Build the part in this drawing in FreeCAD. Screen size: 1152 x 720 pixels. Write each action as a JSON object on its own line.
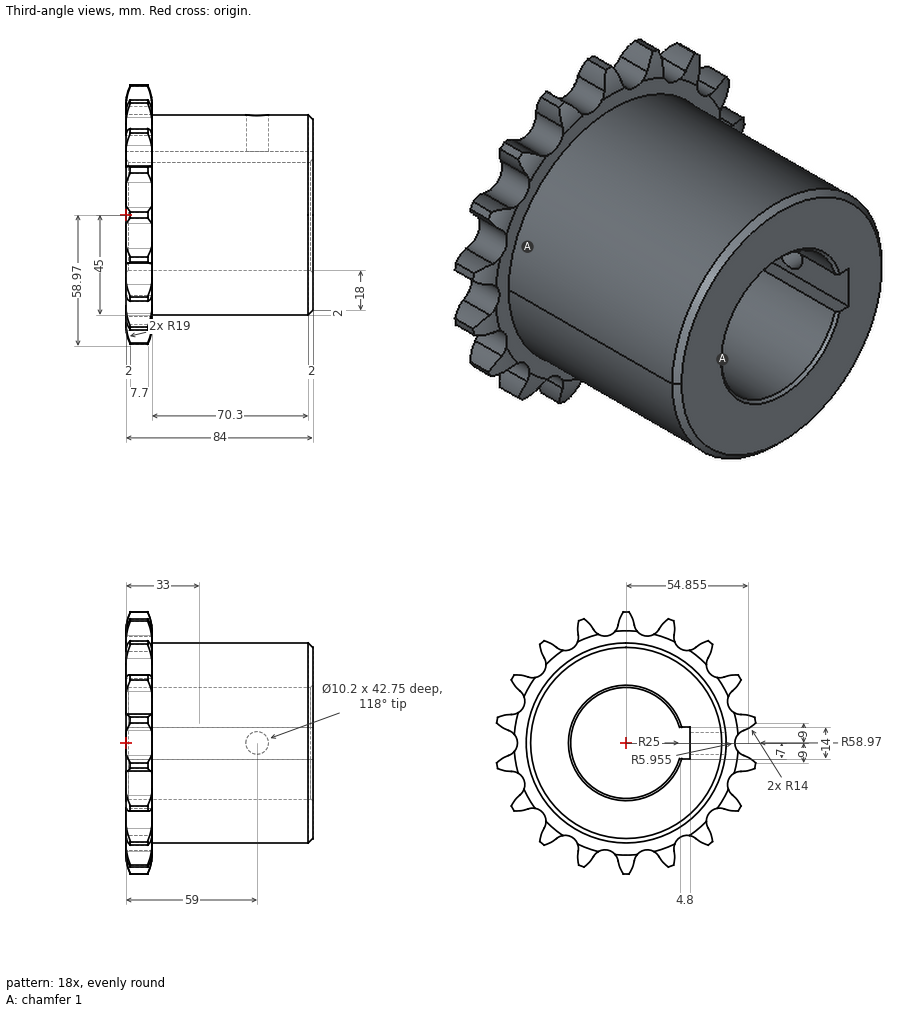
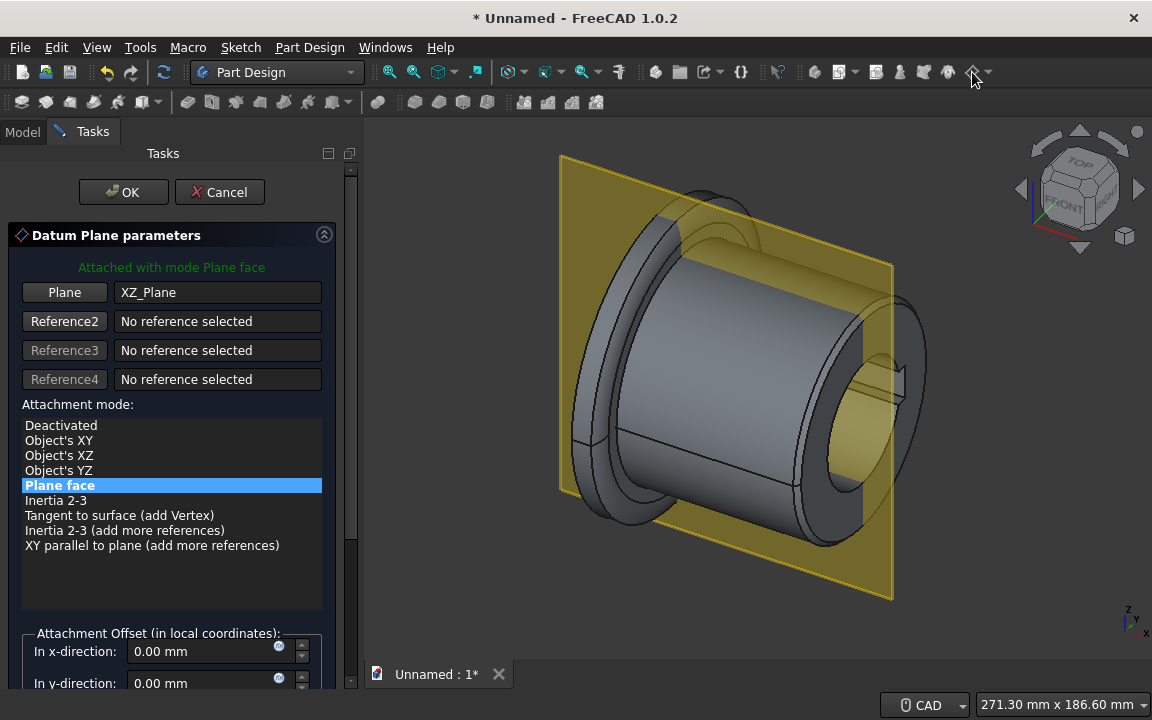
{"action": "scroll", "coordinate": [351, 426], "scroll_direction": "down", "scroll_amount": 2}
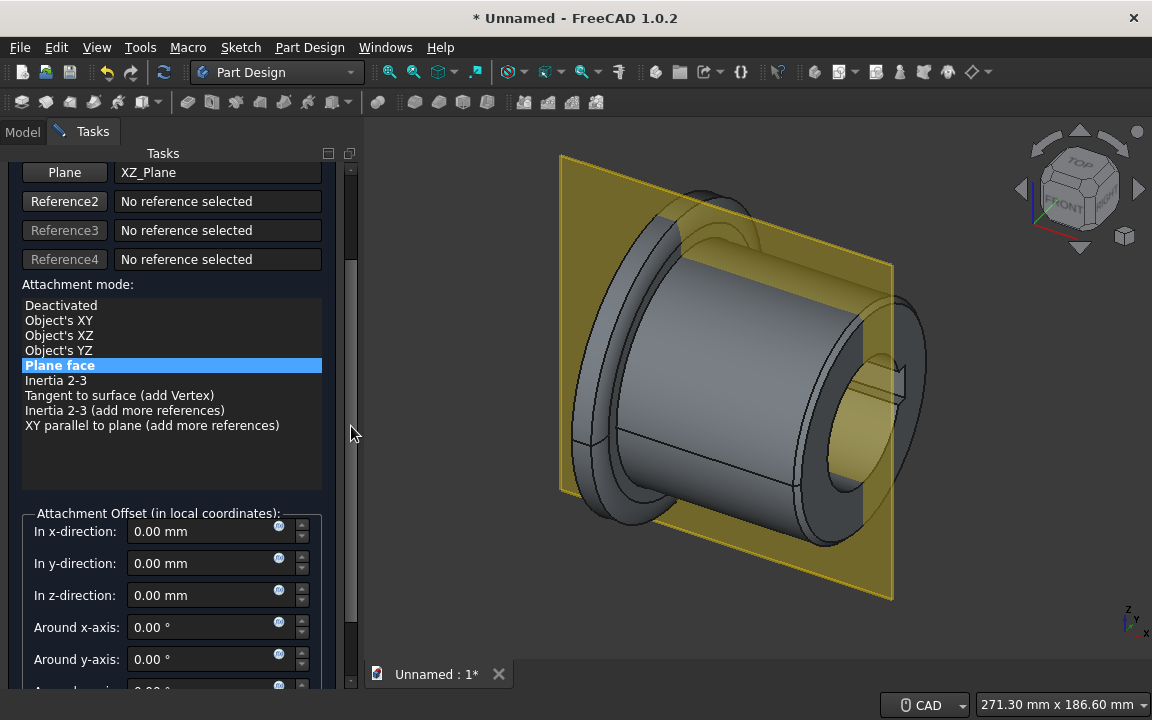
{"action": "triple_click", "coordinate": [210, 595]}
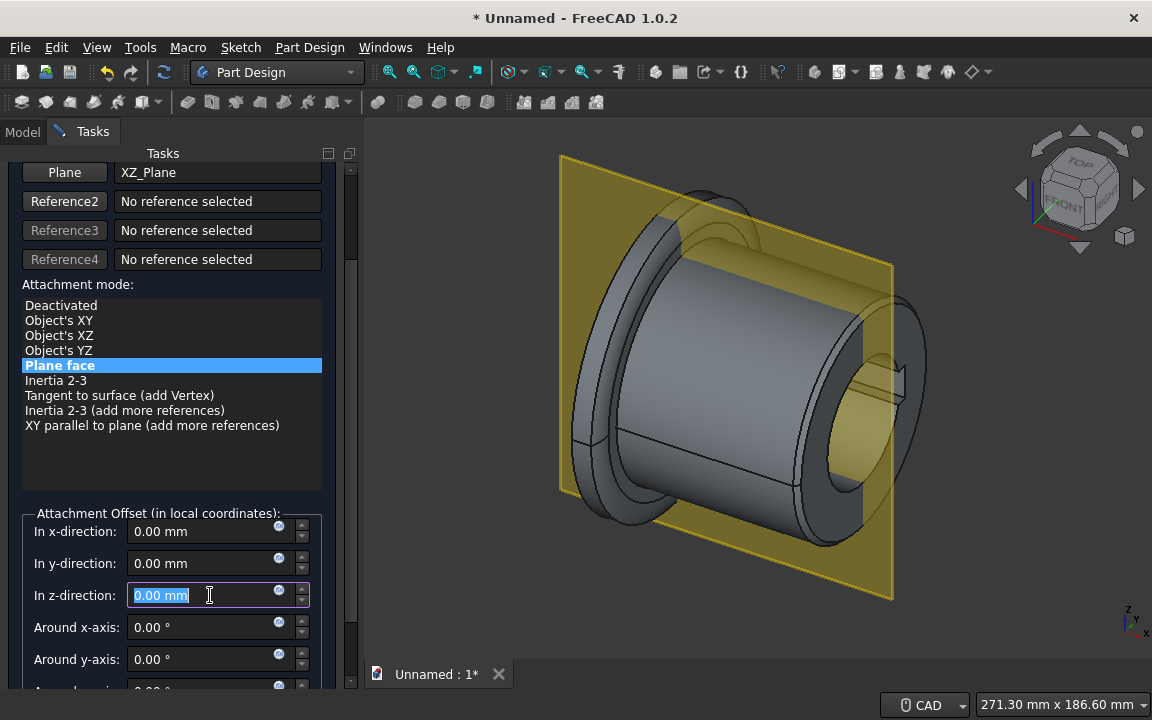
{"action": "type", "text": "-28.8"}
{"action": "key", "text": "Tab"}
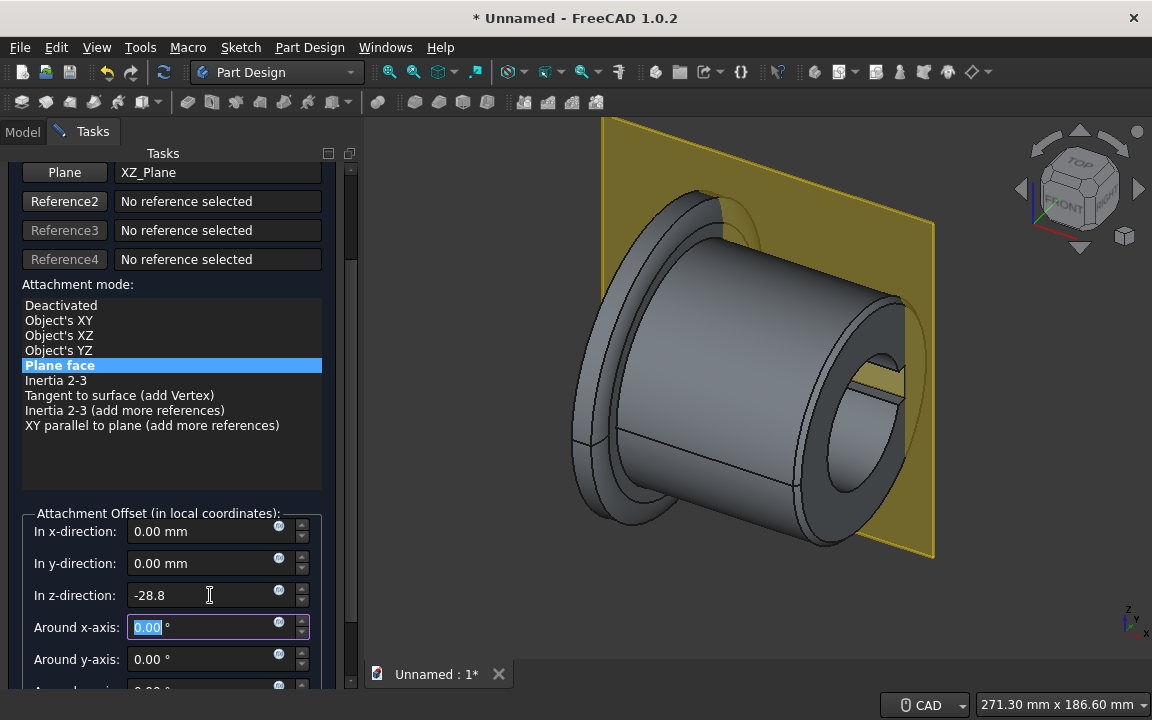
{"action": "scroll", "coordinate": [351, 426], "scroll_direction": "up", "scroll_amount": 3}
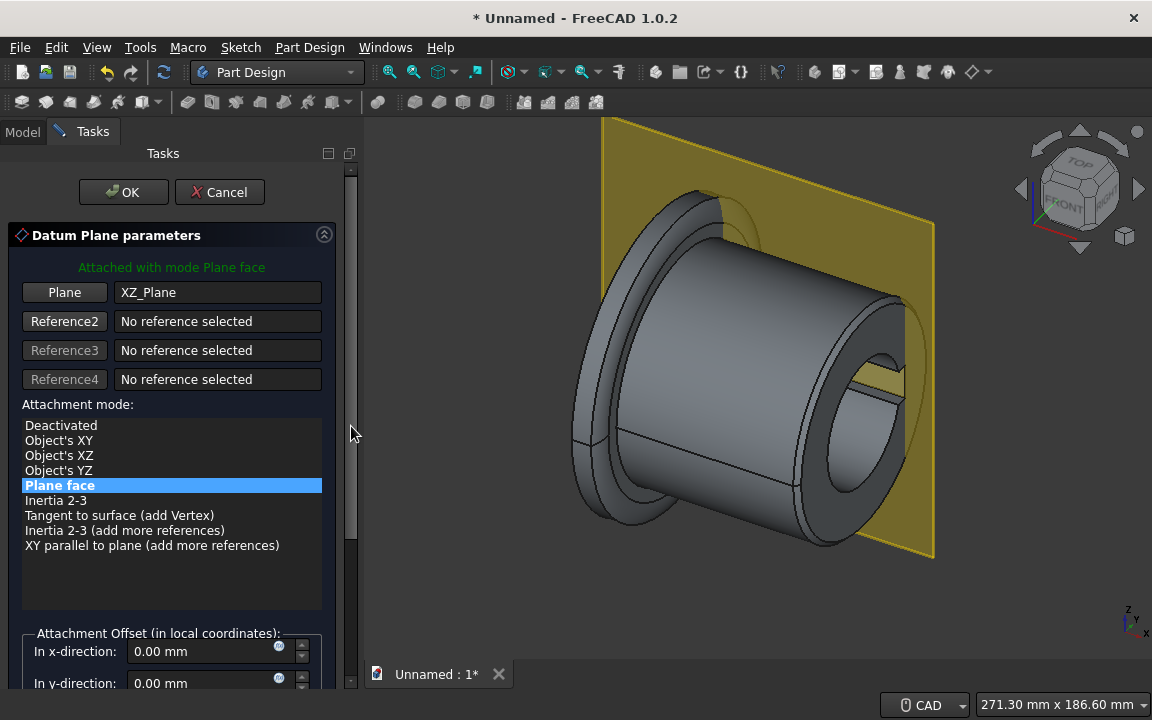
{"action": "left_click", "coordinate": [124, 192]}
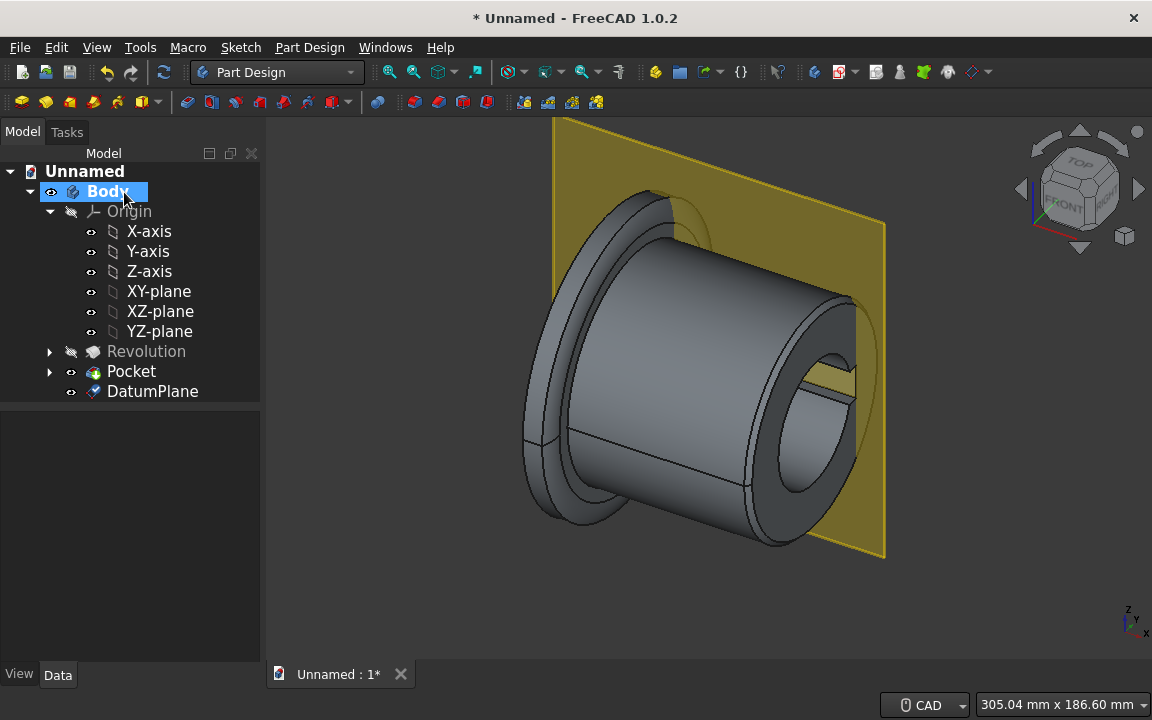
{"action": "left_click", "coordinate": [116, 392]}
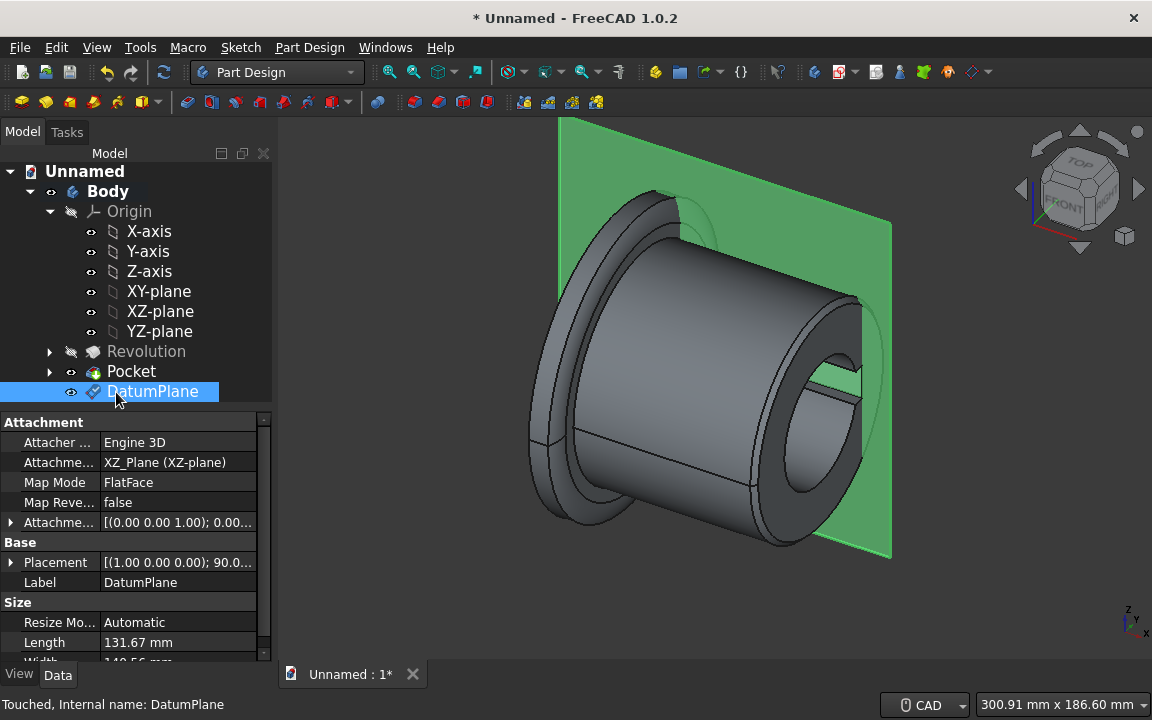
{"action": "left_click", "coordinate": [840, 72]}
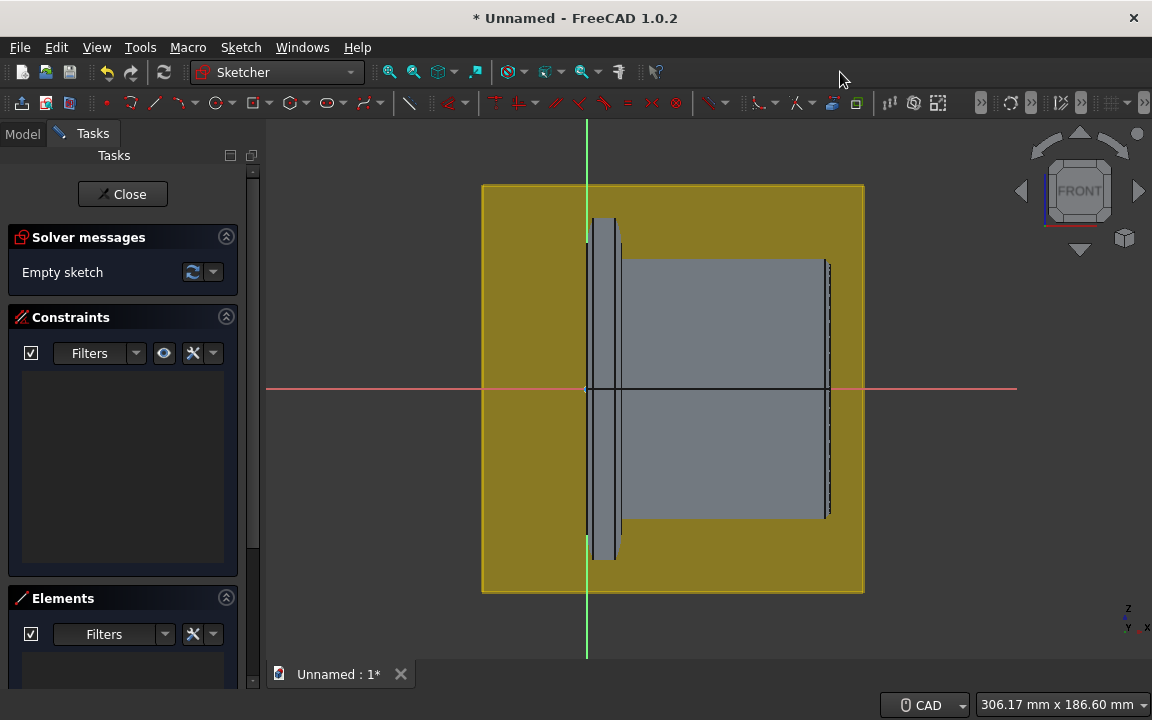
{"action": "left_click", "coordinate": [70, 104]}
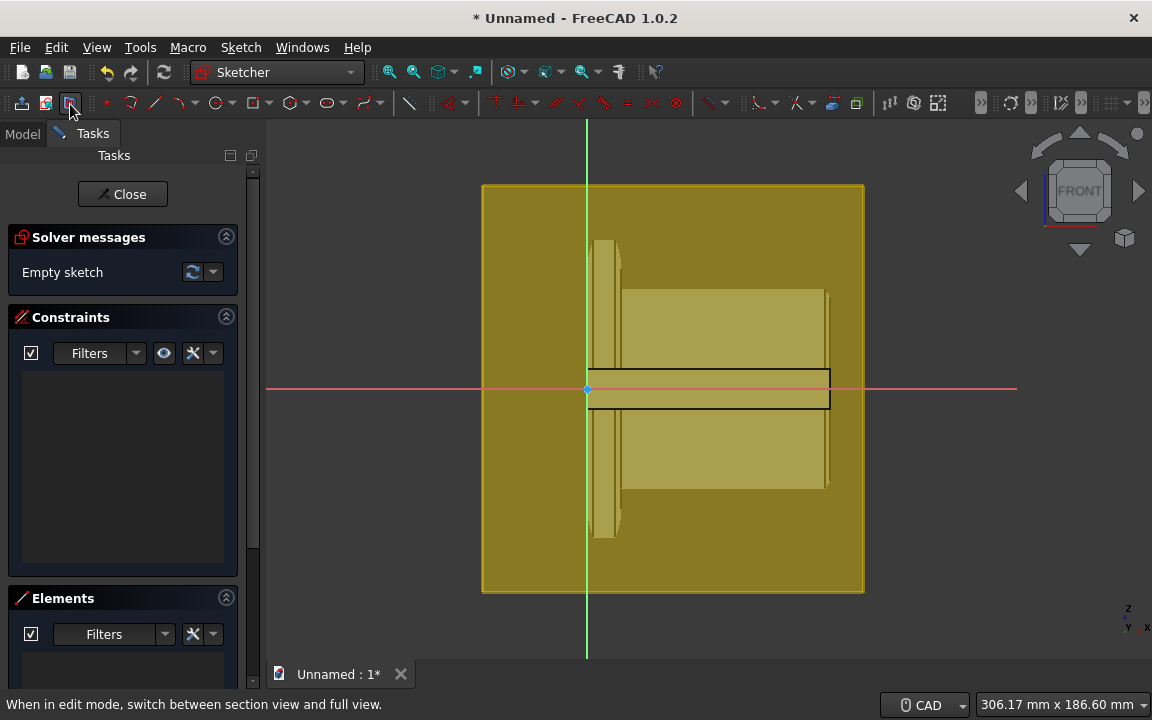
{"action": "scroll", "coordinate": [770, 389], "scroll_direction": "up", "scroll_amount": 12}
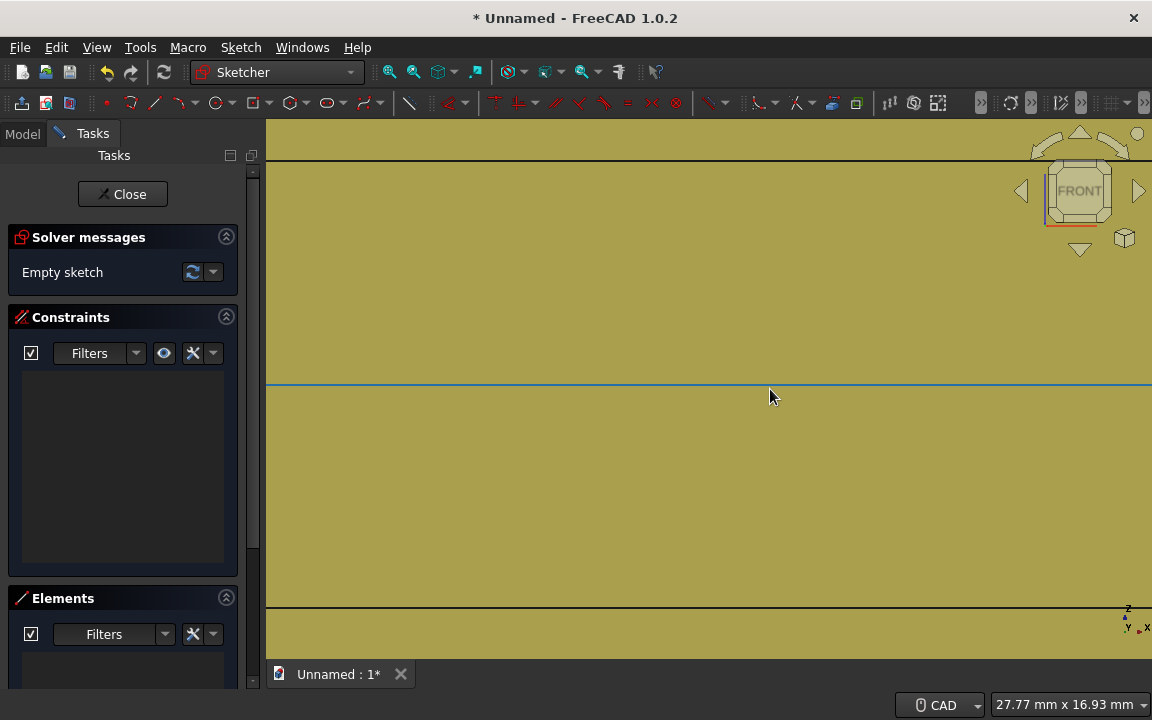
{"action": "key", "text": "g c"}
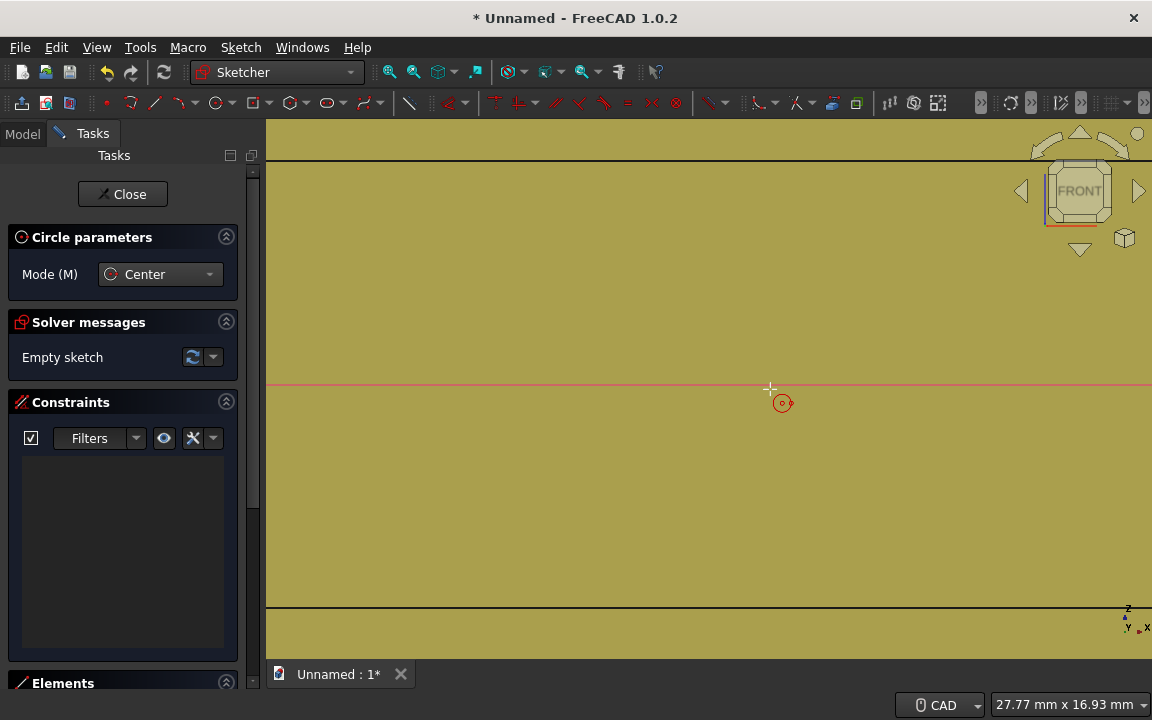
{"action": "left_click", "coordinate": [634, 385]}
{"action": "left_click", "coordinate": [749, 270]}
{"action": "key", "text": "Escape"}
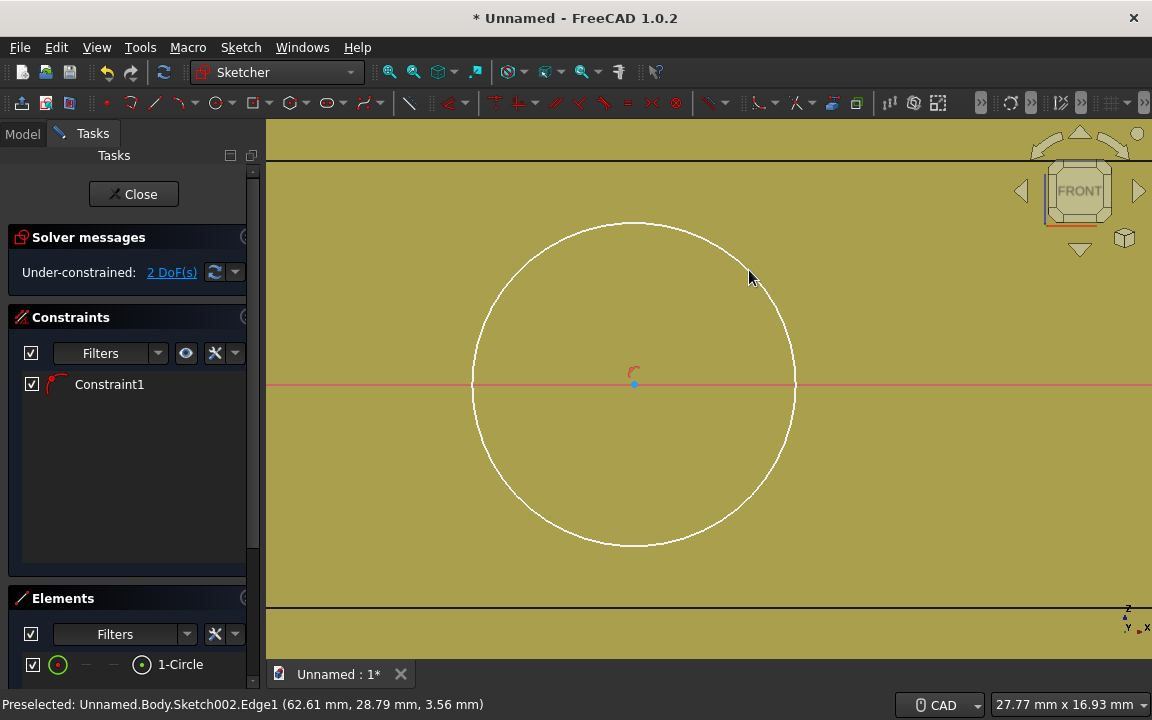
{"action": "left_click", "coordinate": [448, 104]}